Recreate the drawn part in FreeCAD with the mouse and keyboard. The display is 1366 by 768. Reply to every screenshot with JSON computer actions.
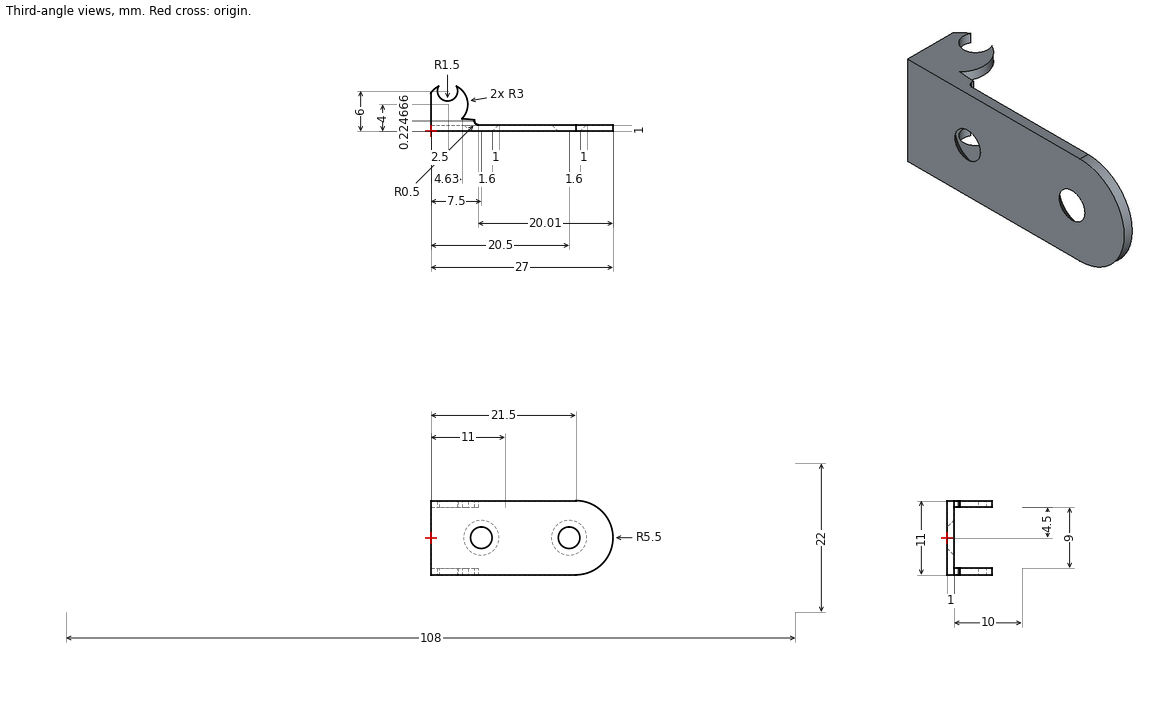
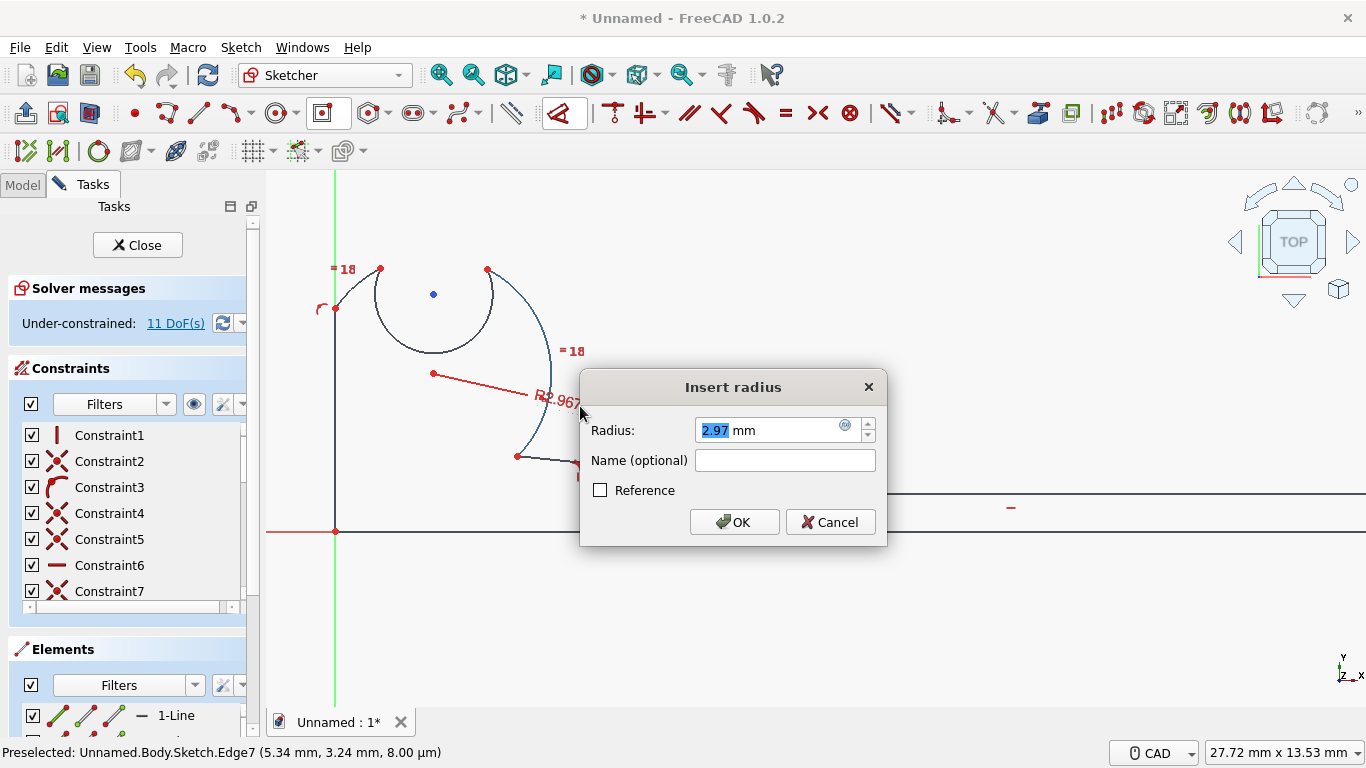
{"action": "type", "text": "3"}
{"action": "key", "text": "Return"}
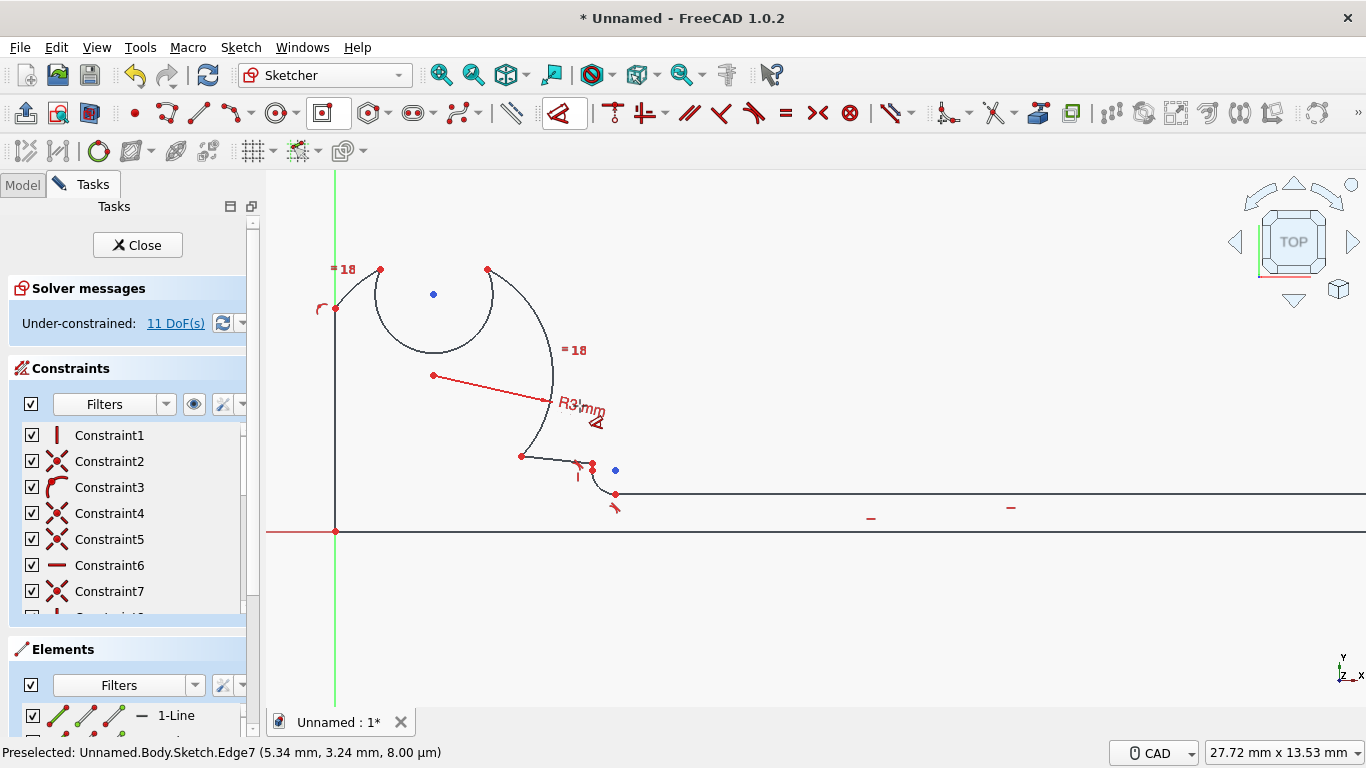
{"action": "left_click", "coordinate": [391, 335]}
{"action": "left_click", "coordinate": [368, 357]}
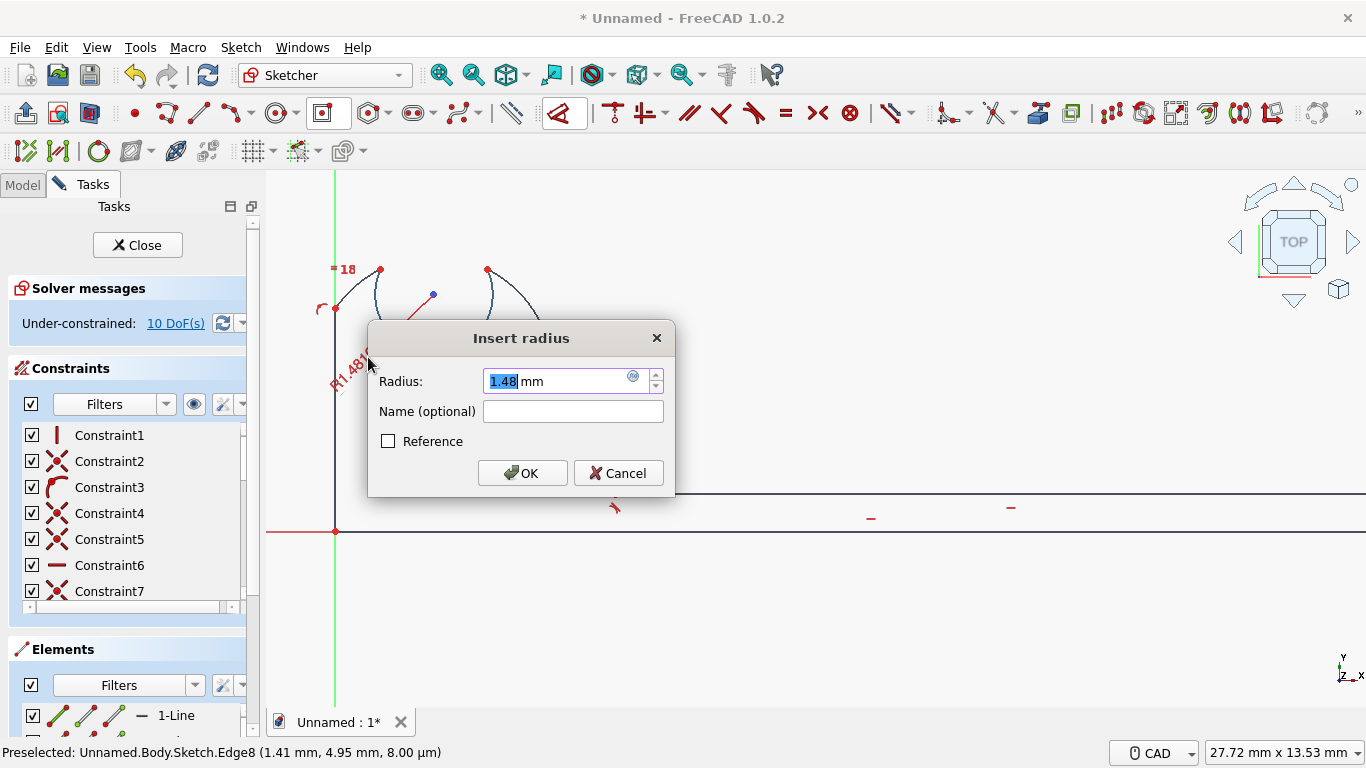
{"action": "type", "text": "1.5"}
{"action": "key", "text": "Return"}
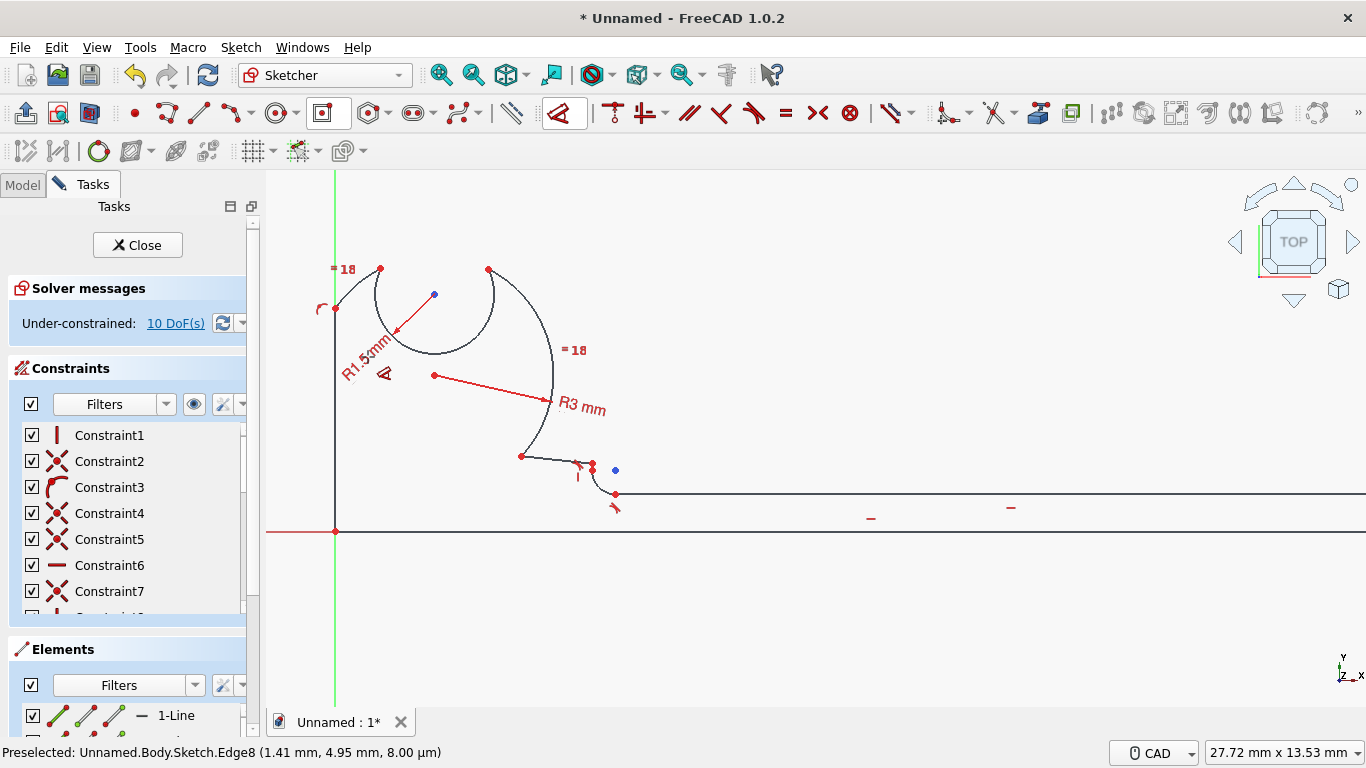
{"action": "scroll", "coordinate": [595, 481], "scroll_direction": "up", "scroll_amount": 4}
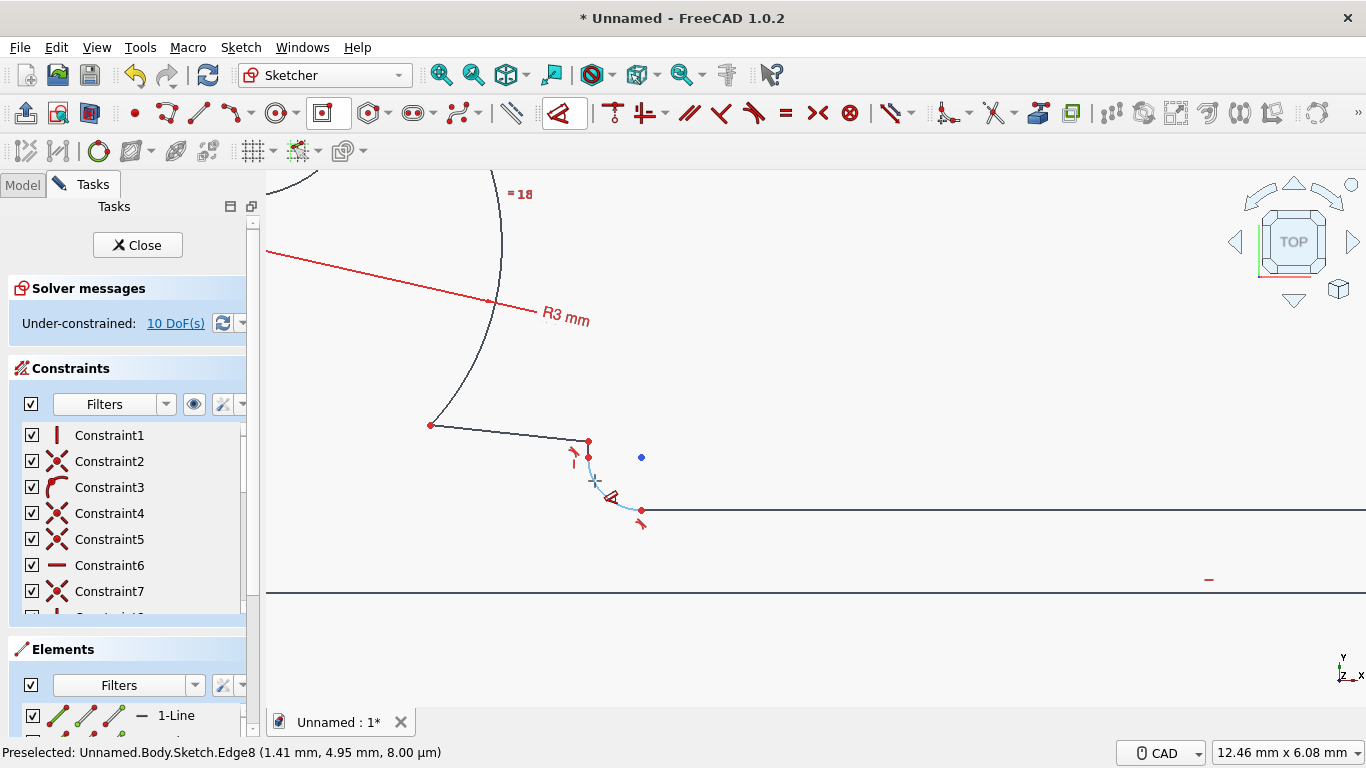
{"action": "left_click", "coordinate": [594, 481]}
{"action": "left_click", "coordinate": [565, 495]}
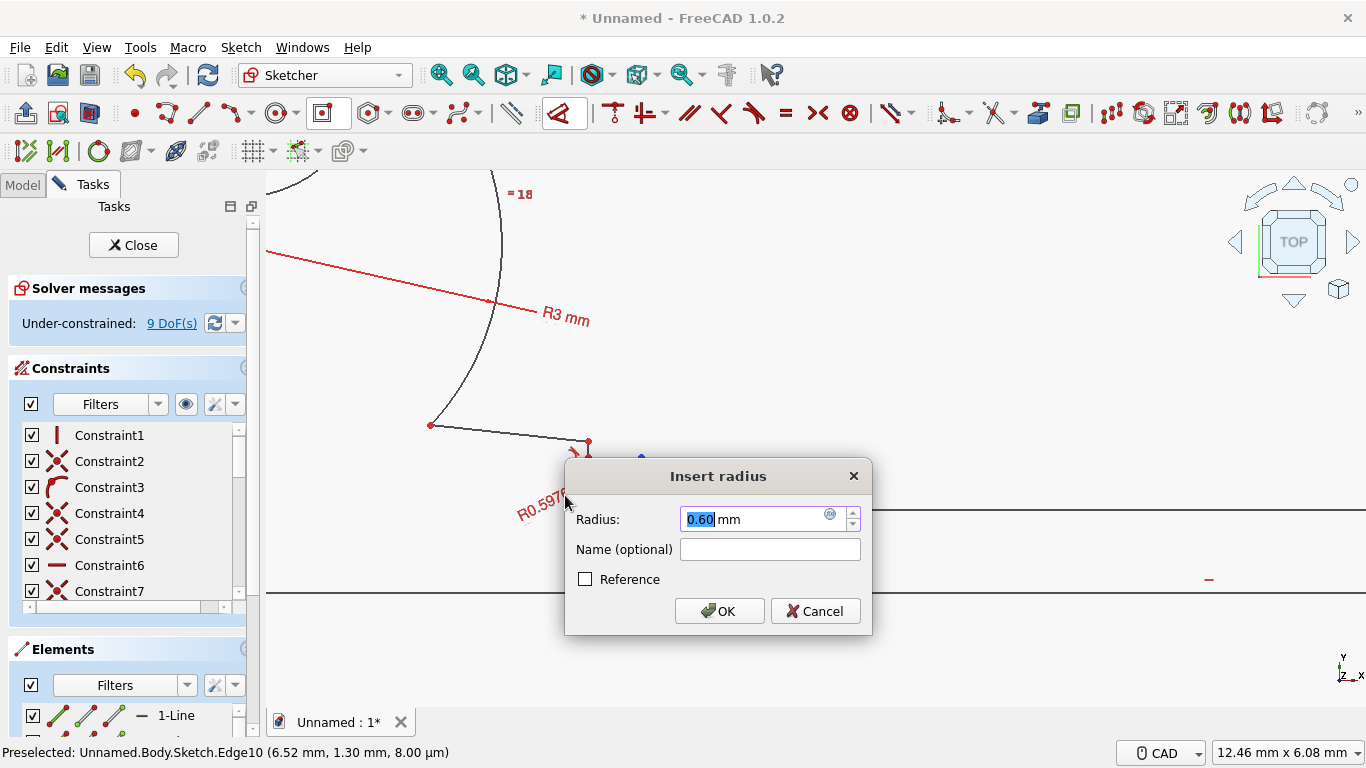
{"action": "type", "text": "0.5"}
{"action": "key", "text": "Return"}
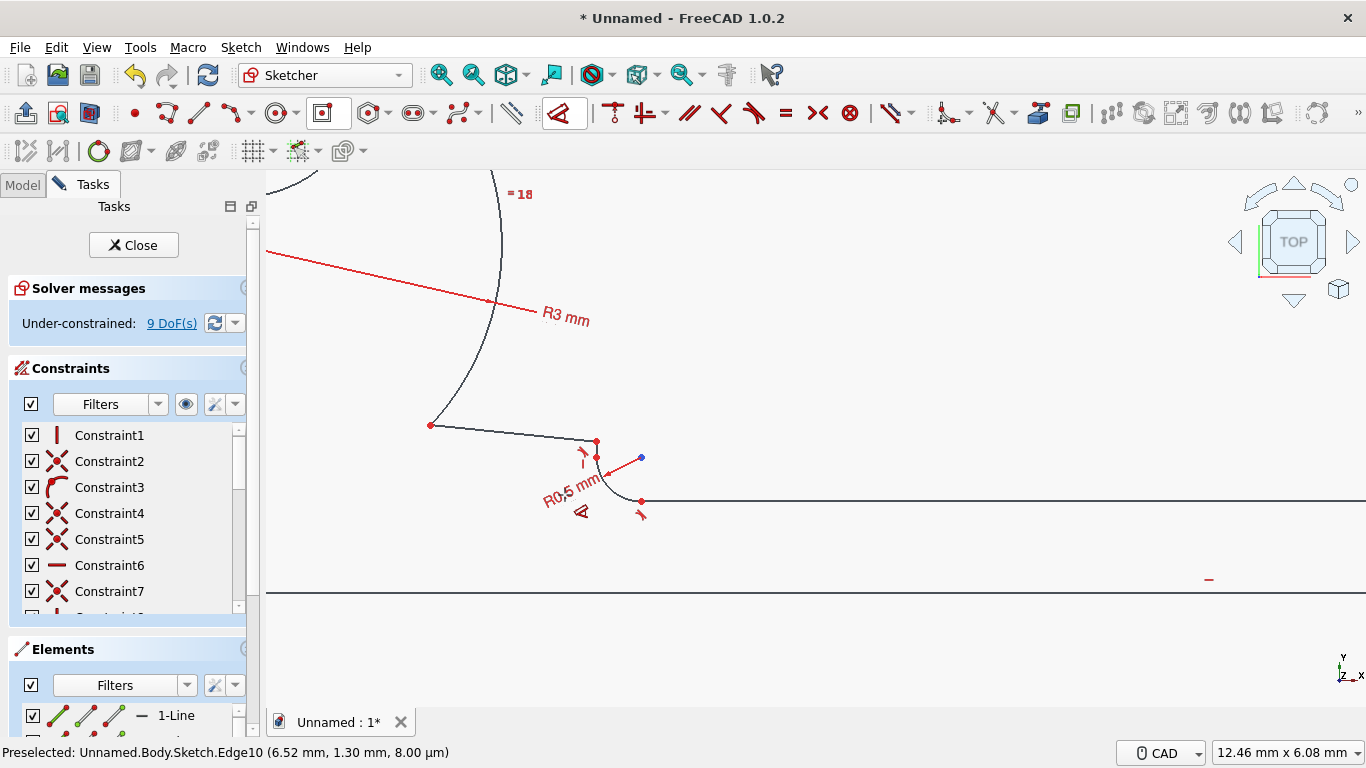
{"action": "scroll", "coordinate": [596, 485], "scroll_direction": "down", "scroll_amount": 7}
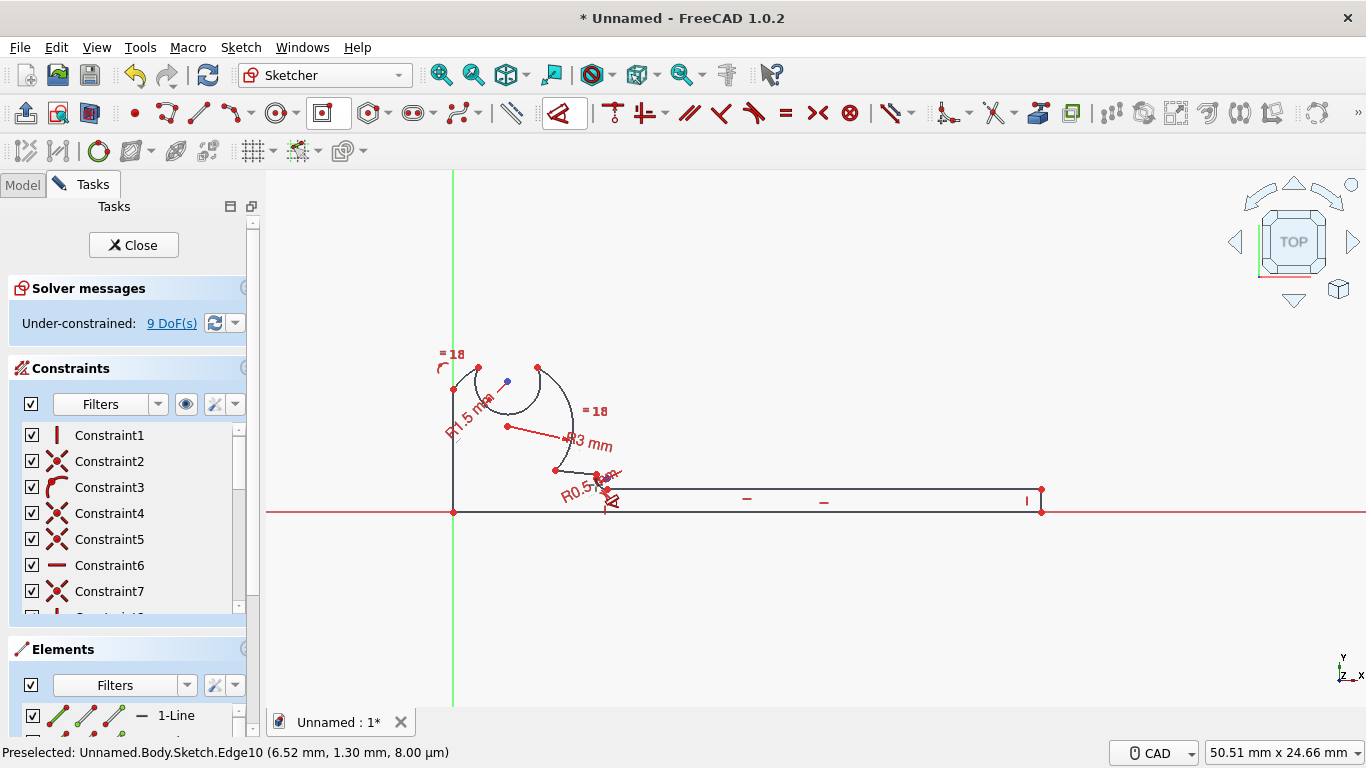
{"action": "scroll", "coordinate": [1041, 505], "scroll_direction": "up", "scroll_amount": 4}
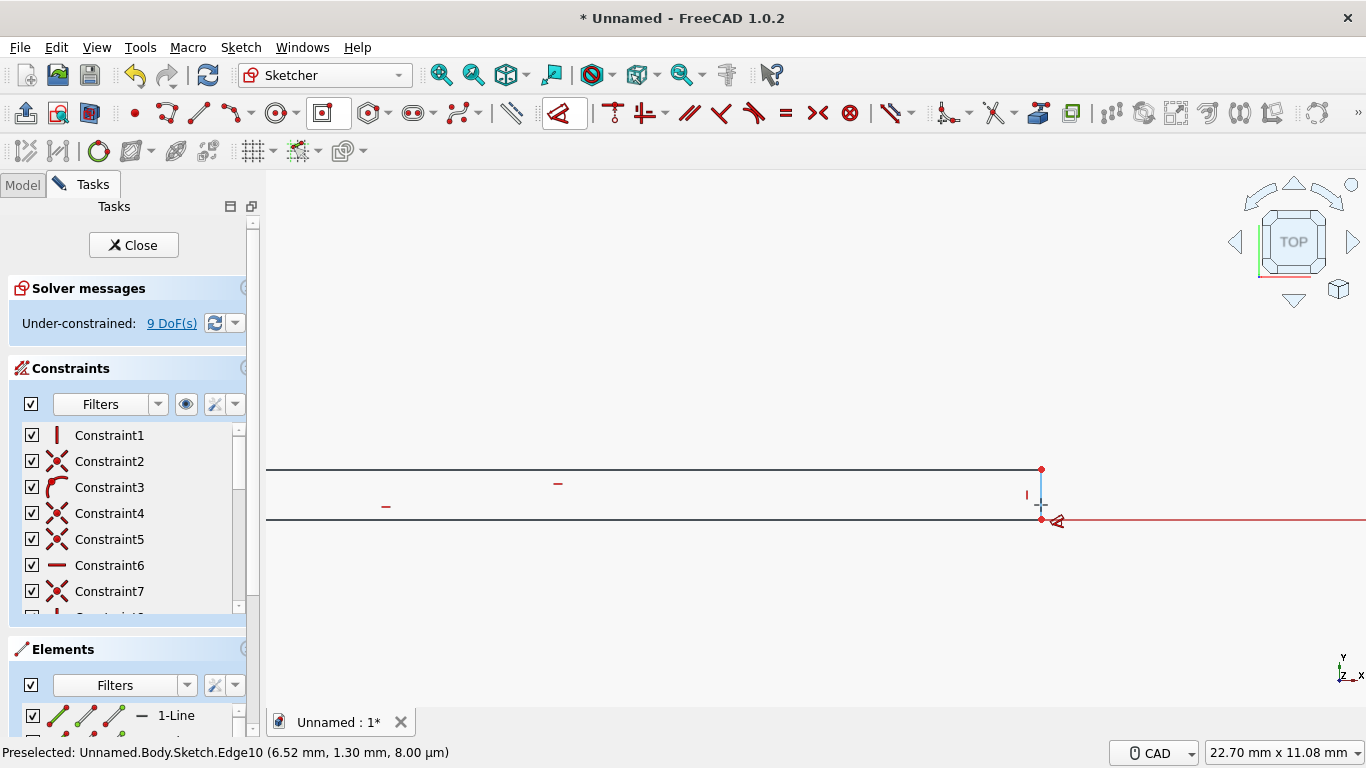
{"action": "left_click", "coordinate": [1041, 505]}
{"action": "left_click", "coordinate": [1075, 495]}